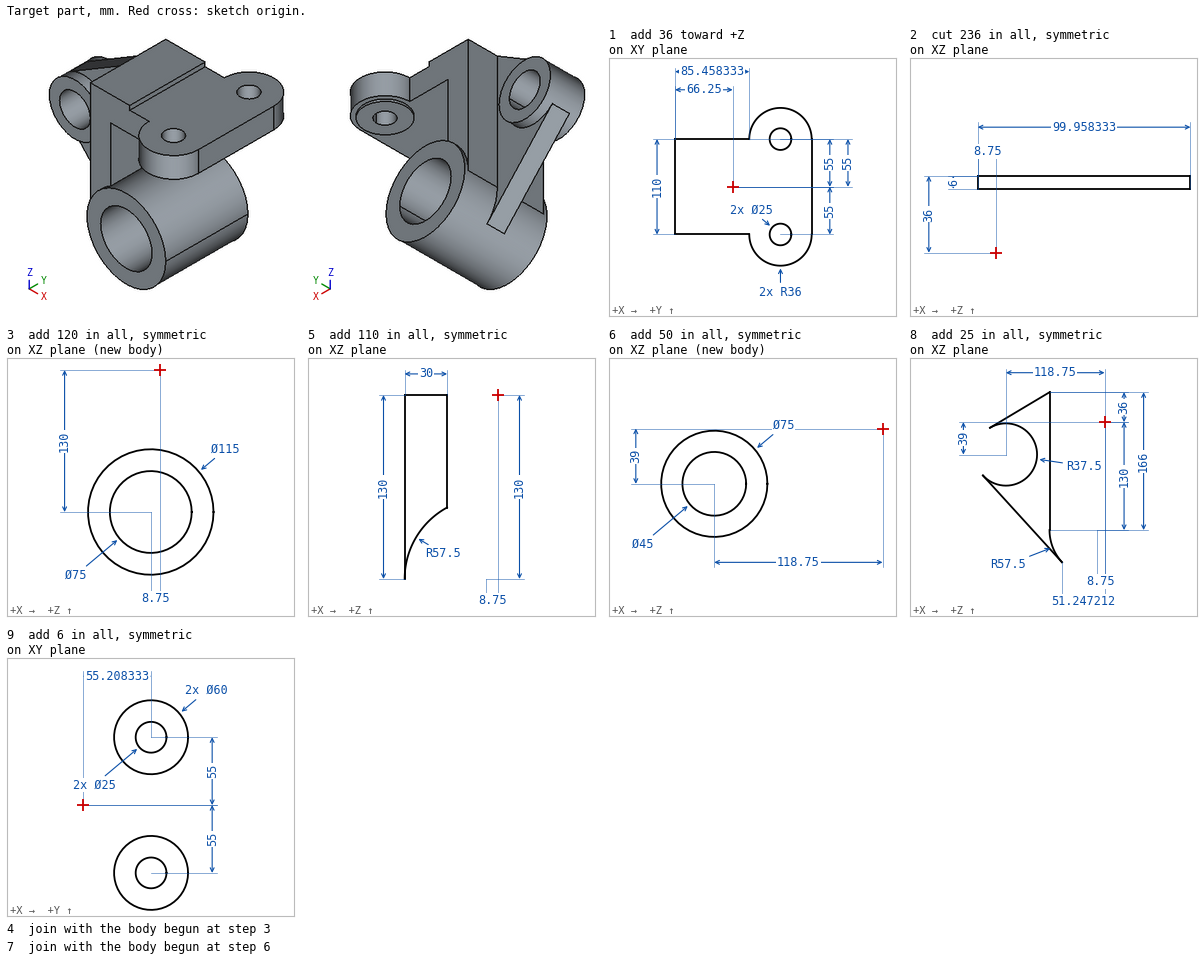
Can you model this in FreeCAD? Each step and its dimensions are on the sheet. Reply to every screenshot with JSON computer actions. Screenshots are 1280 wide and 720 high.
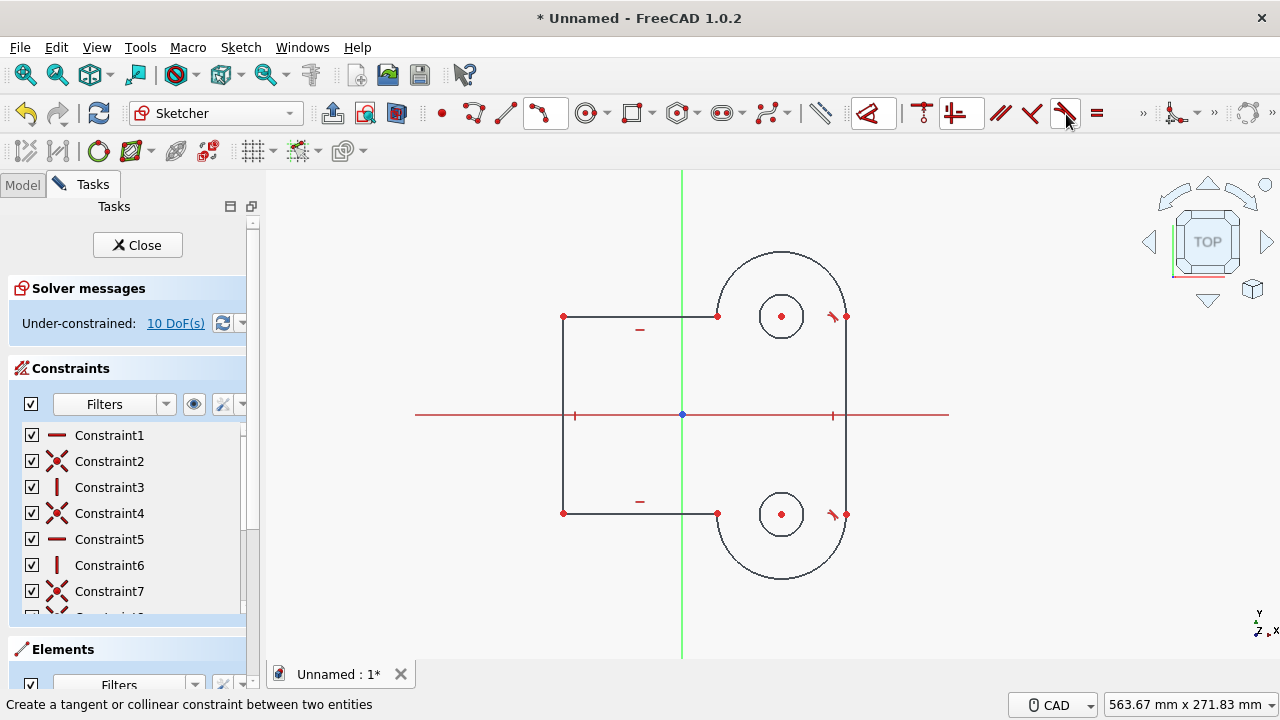
{"action": "left_click", "coordinate": [743, 566]}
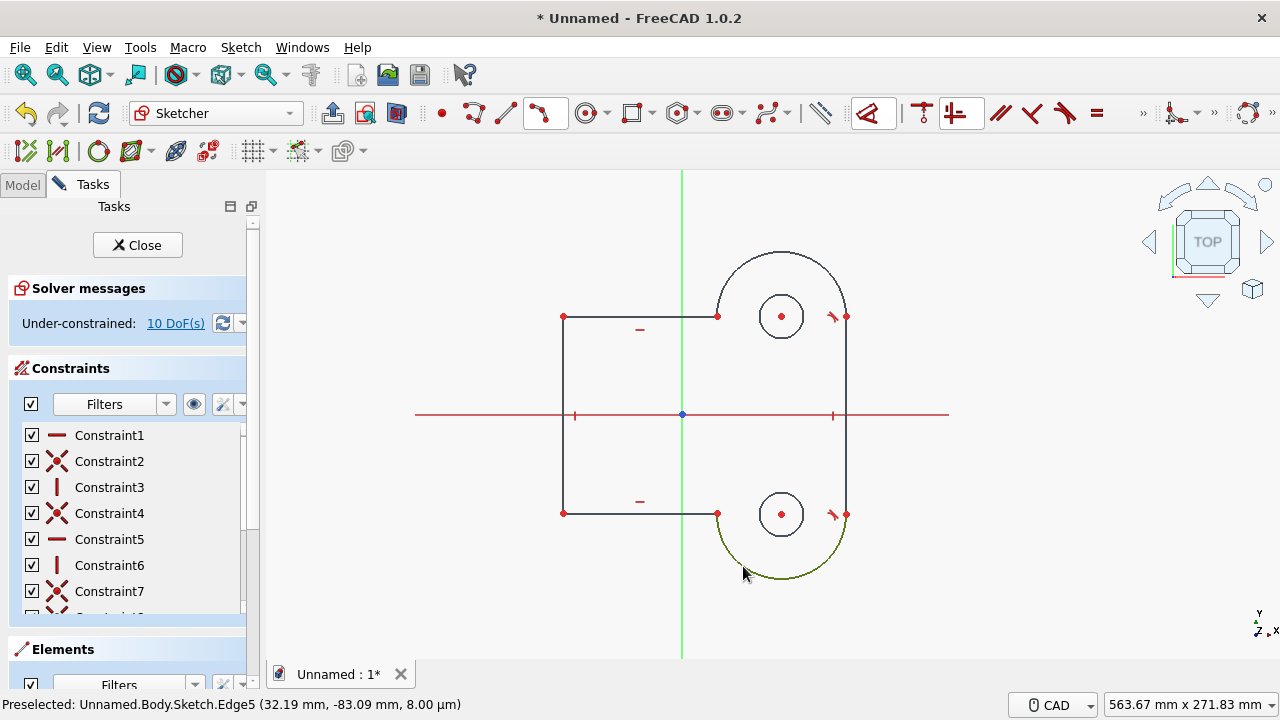
{"action": "left_click", "coordinate": [819, 264]}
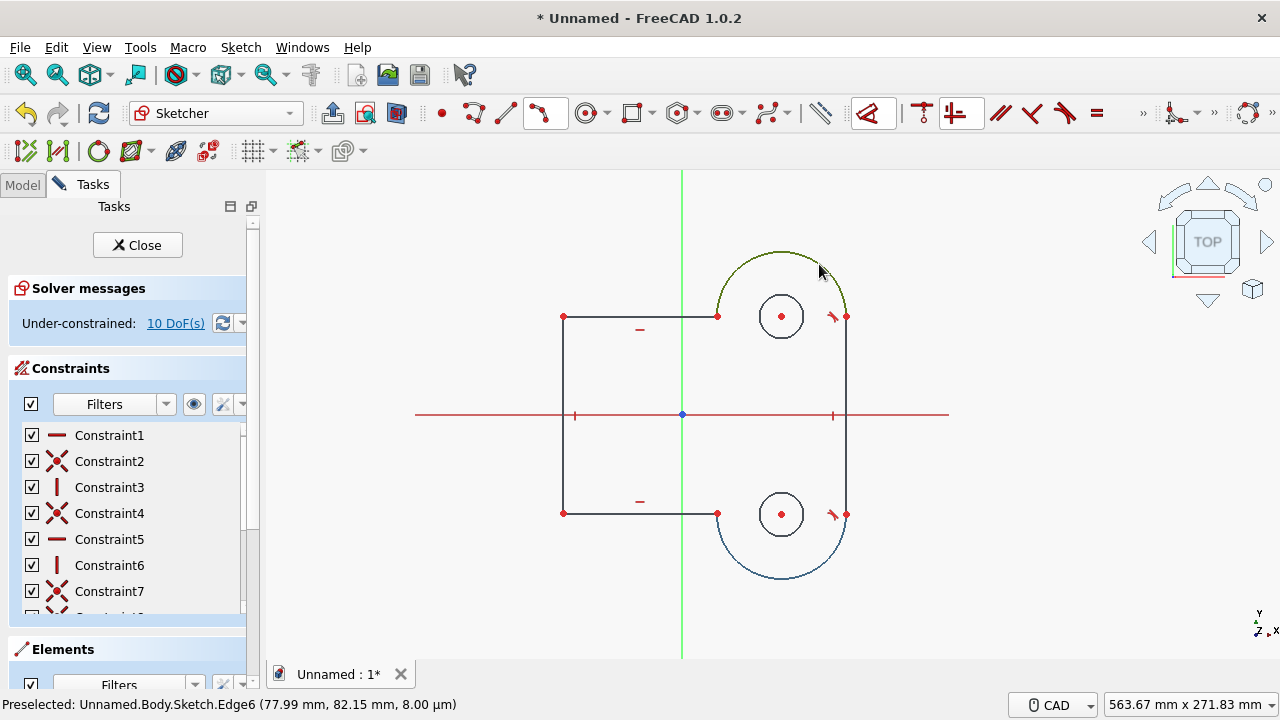
{"action": "key", "text": "e"}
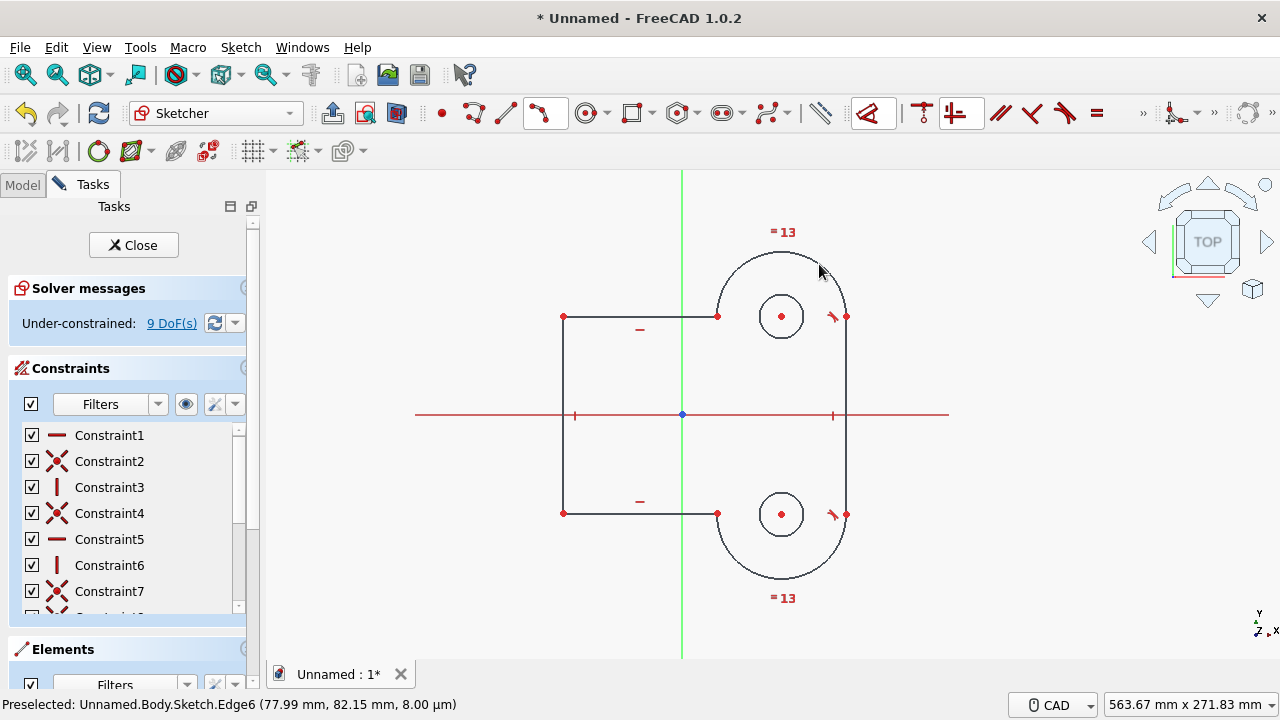
{"action": "left_click", "coordinate": [797, 499]}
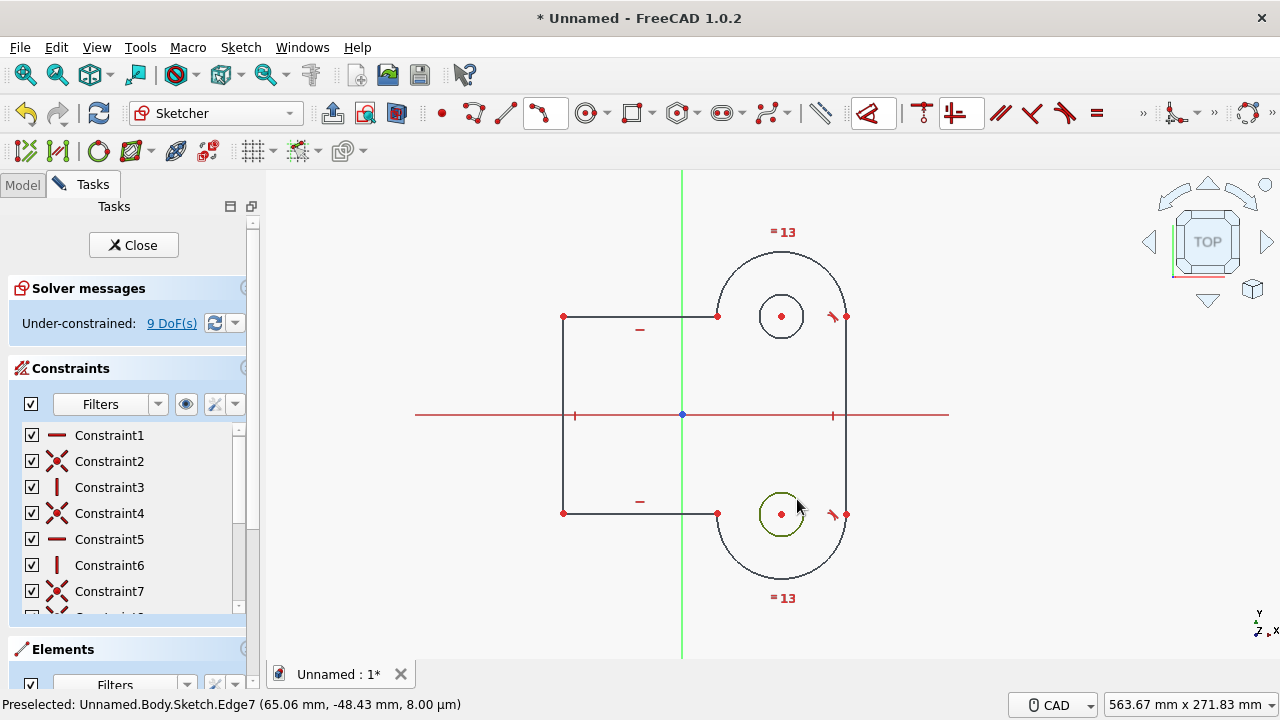
{"action": "left_click", "coordinate": [797, 301]}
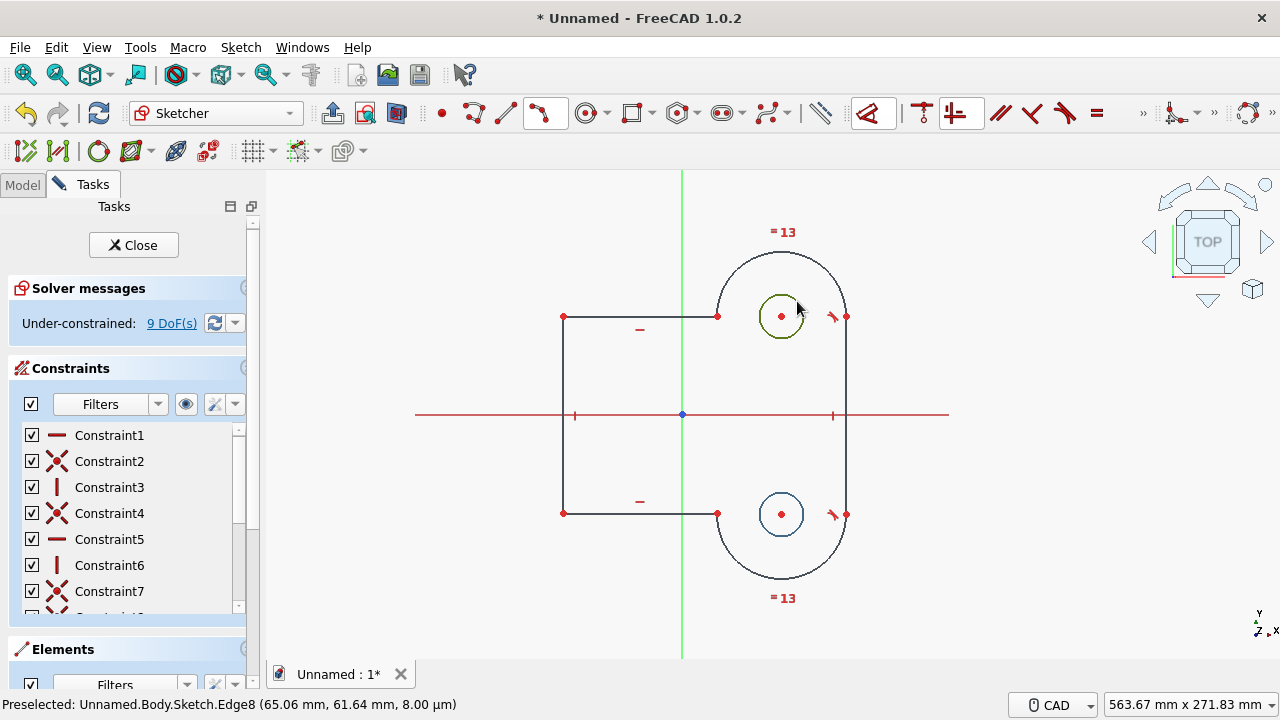
{"action": "left_click", "coordinate": [1098, 114]}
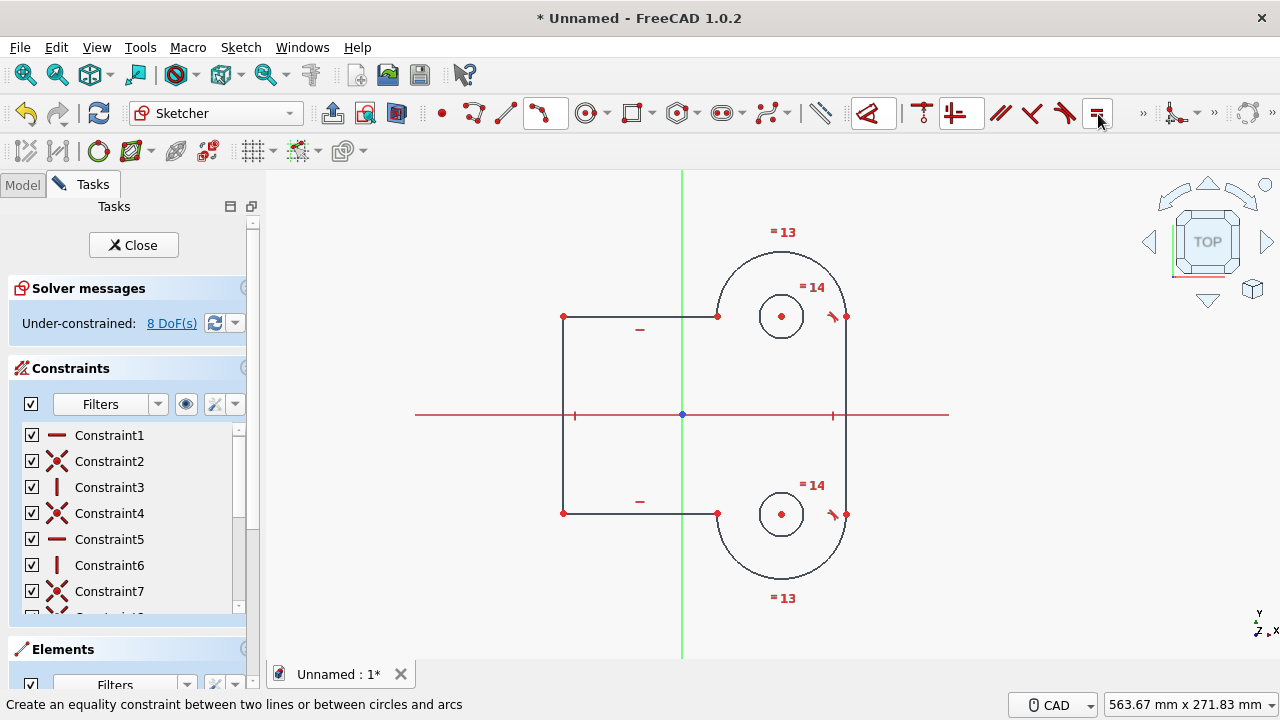
{"action": "left_click", "coordinate": [868, 114]}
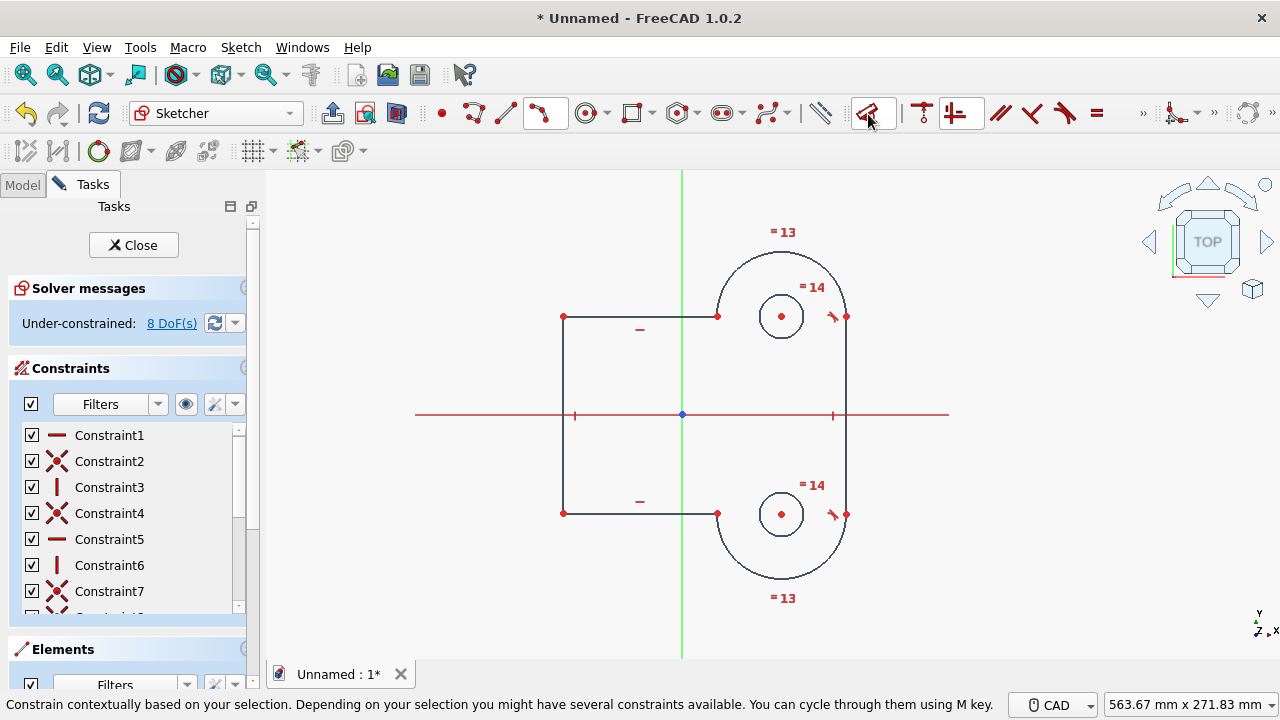
{"action": "left_click", "coordinate": [743, 566]}
{"action": "left_click", "coordinate": [724, 592]}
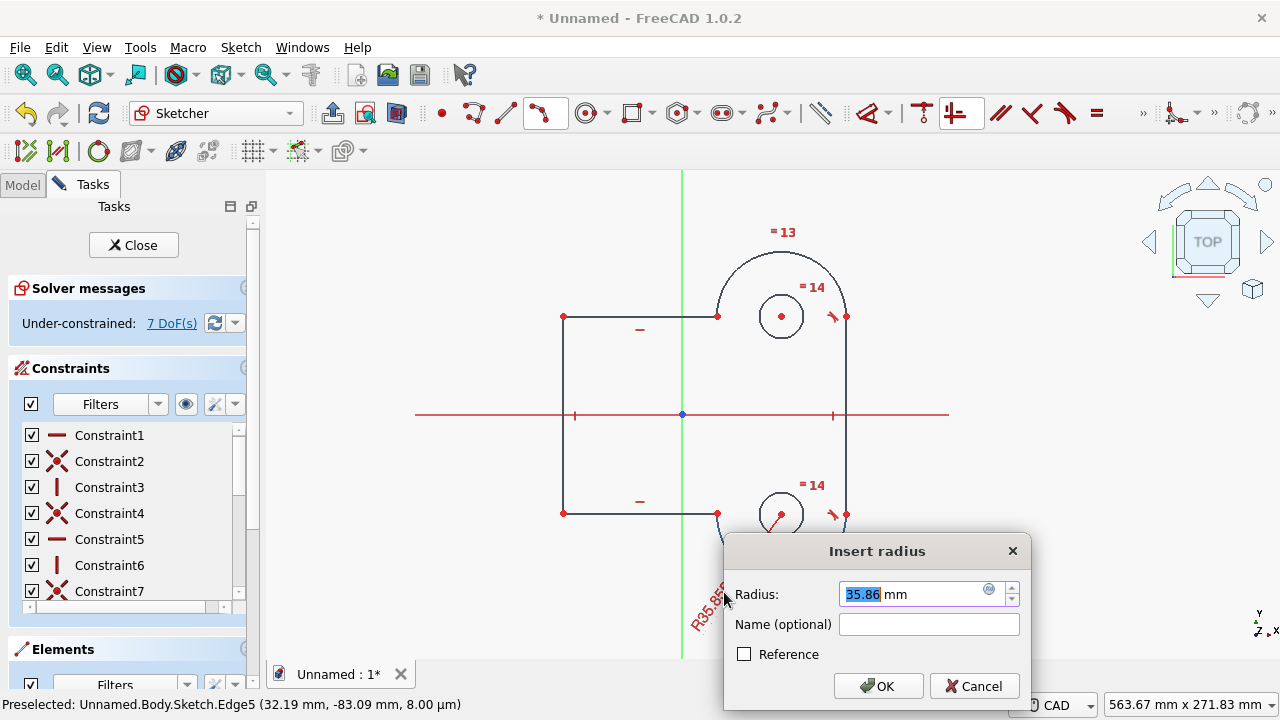
{"action": "type", "text": "36"}
{"action": "key", "text": "Return"}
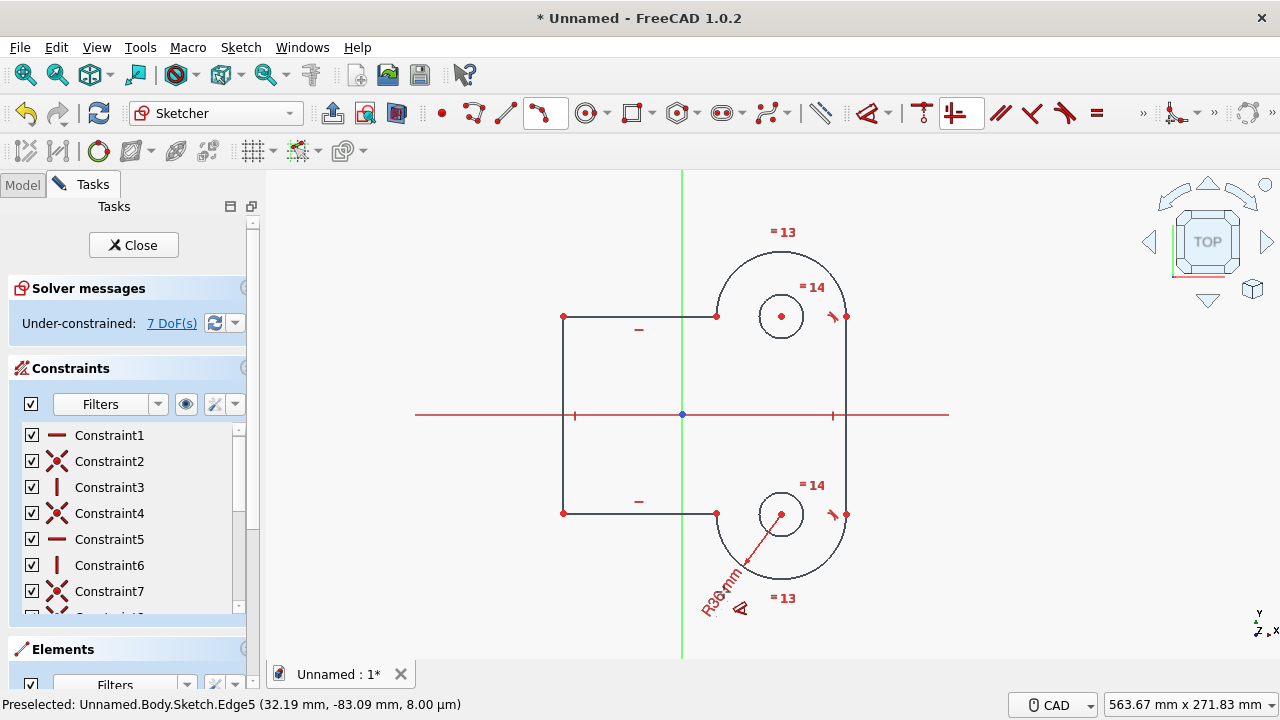
{"action": "left_click", "coordinate": [797, 499]}
{"action": "left_click", "coordinate": [820, 476]}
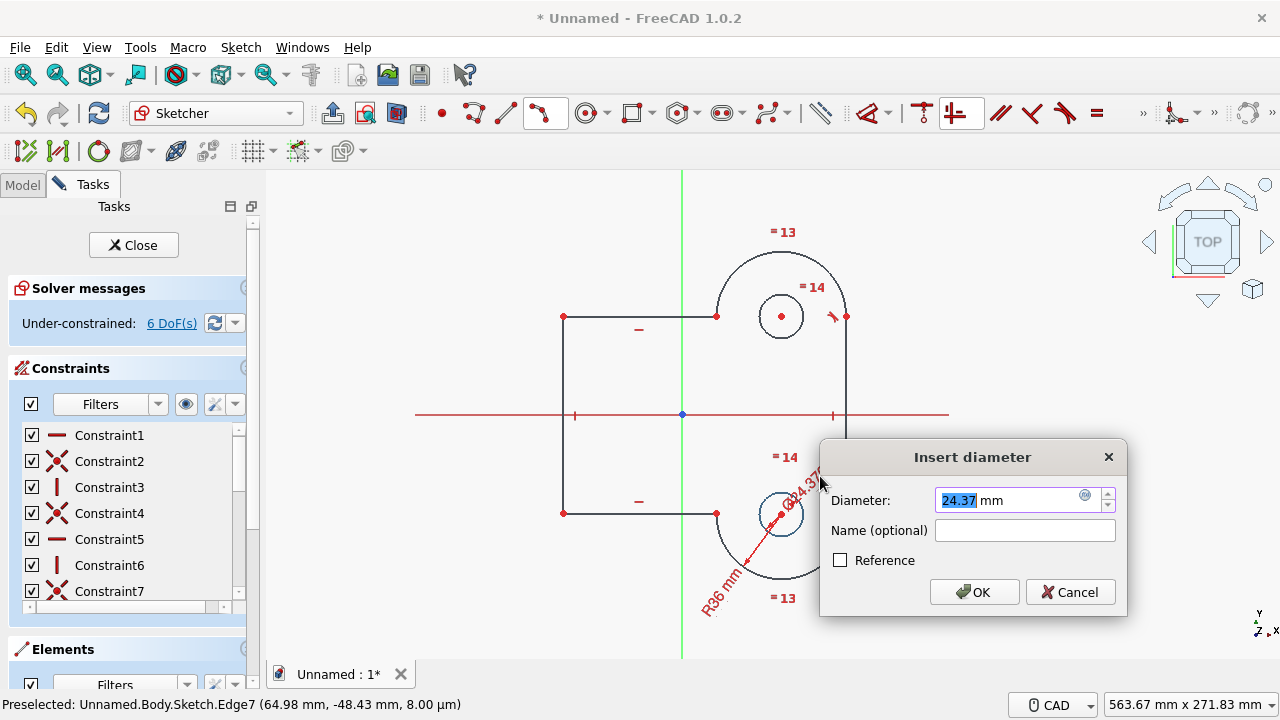
{"action": "type", "text": "25"}
{"action": "key", "text": "Return"}